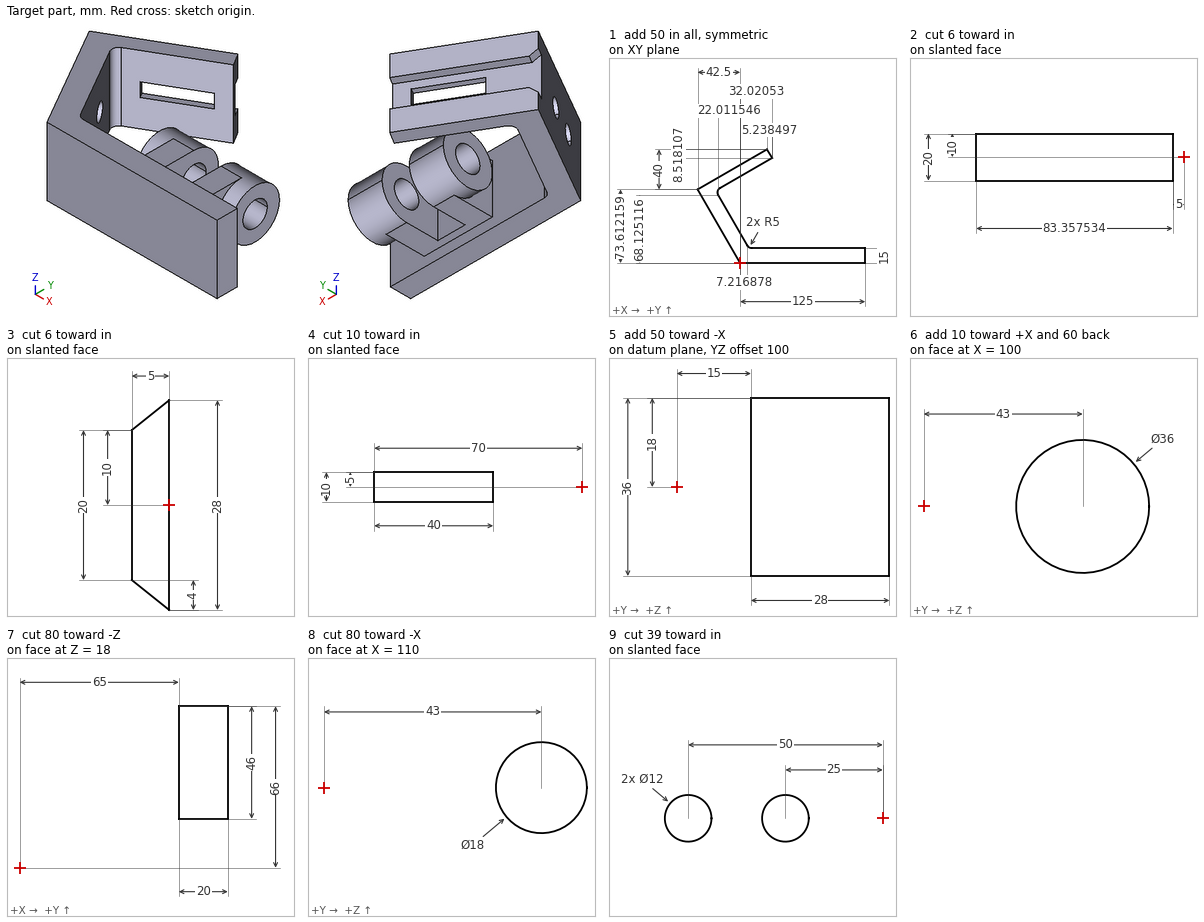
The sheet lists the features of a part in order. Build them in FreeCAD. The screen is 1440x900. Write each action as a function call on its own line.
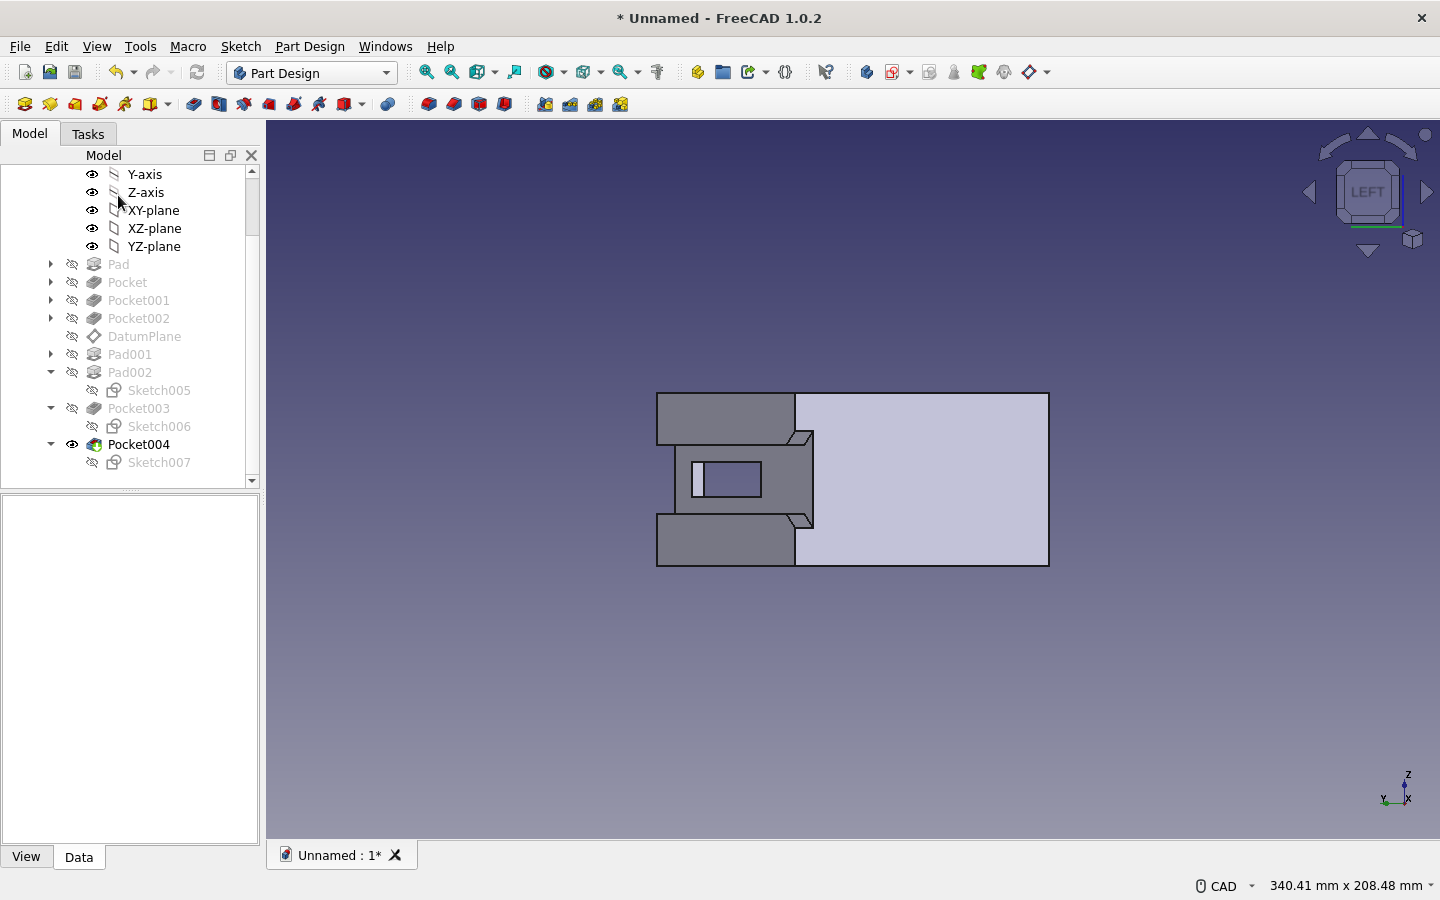
click(958, 478)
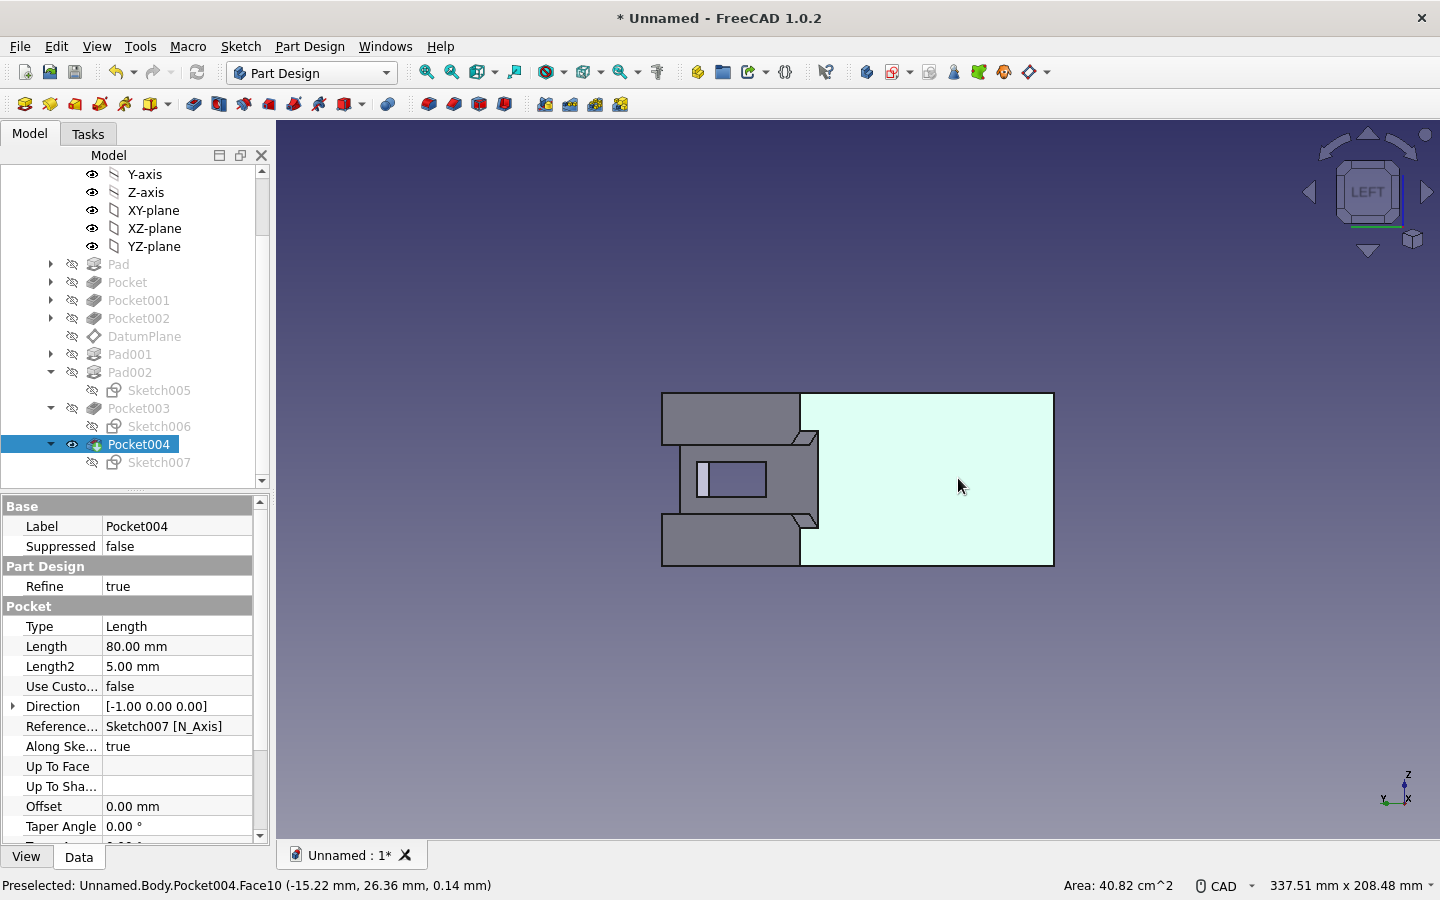
click(892, 72)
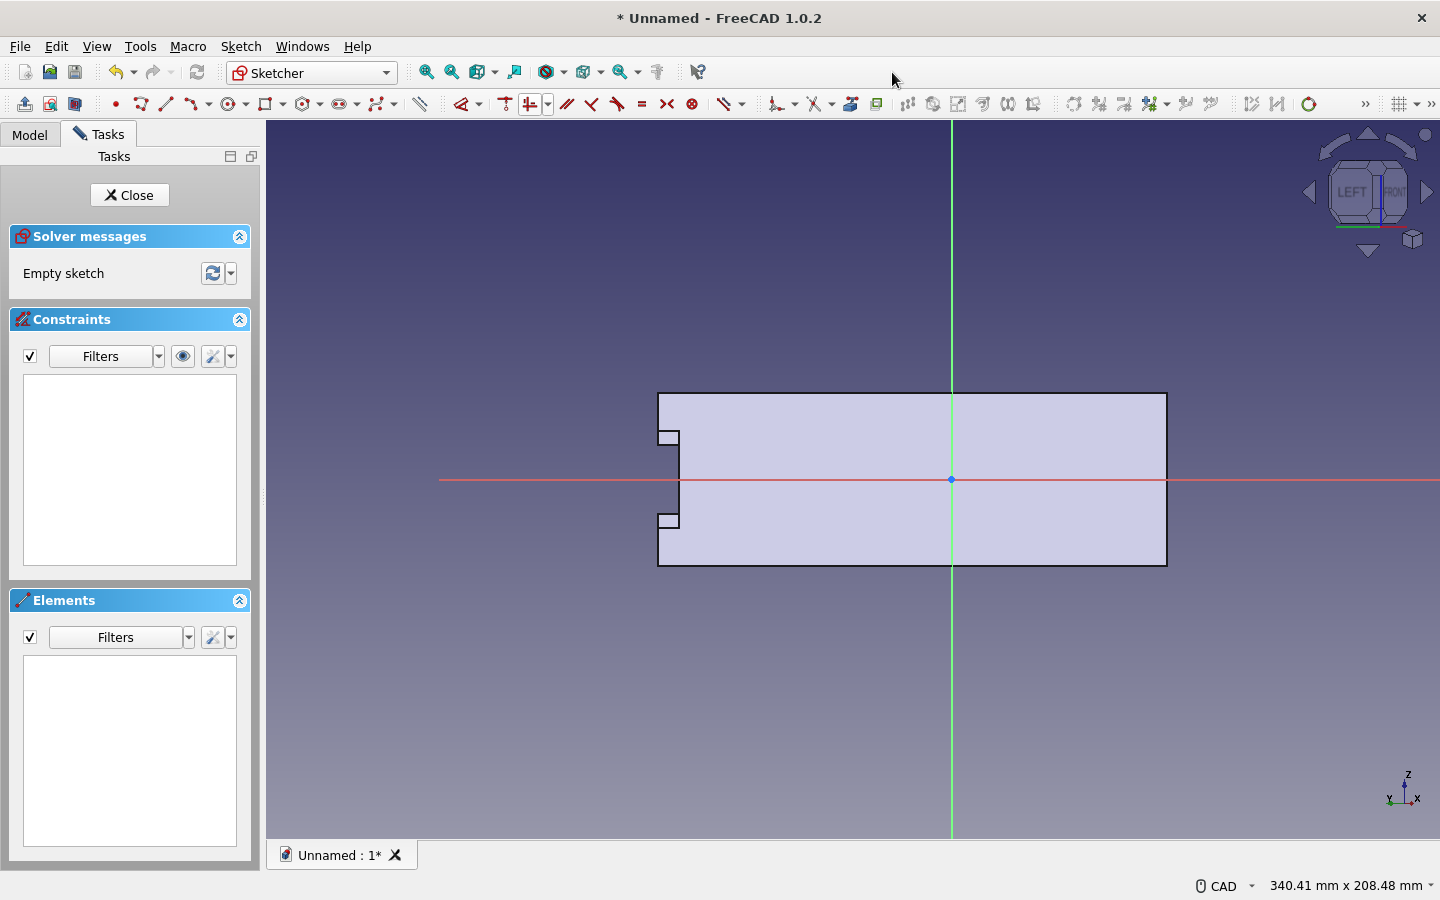
scroll(885, 479, up, 6)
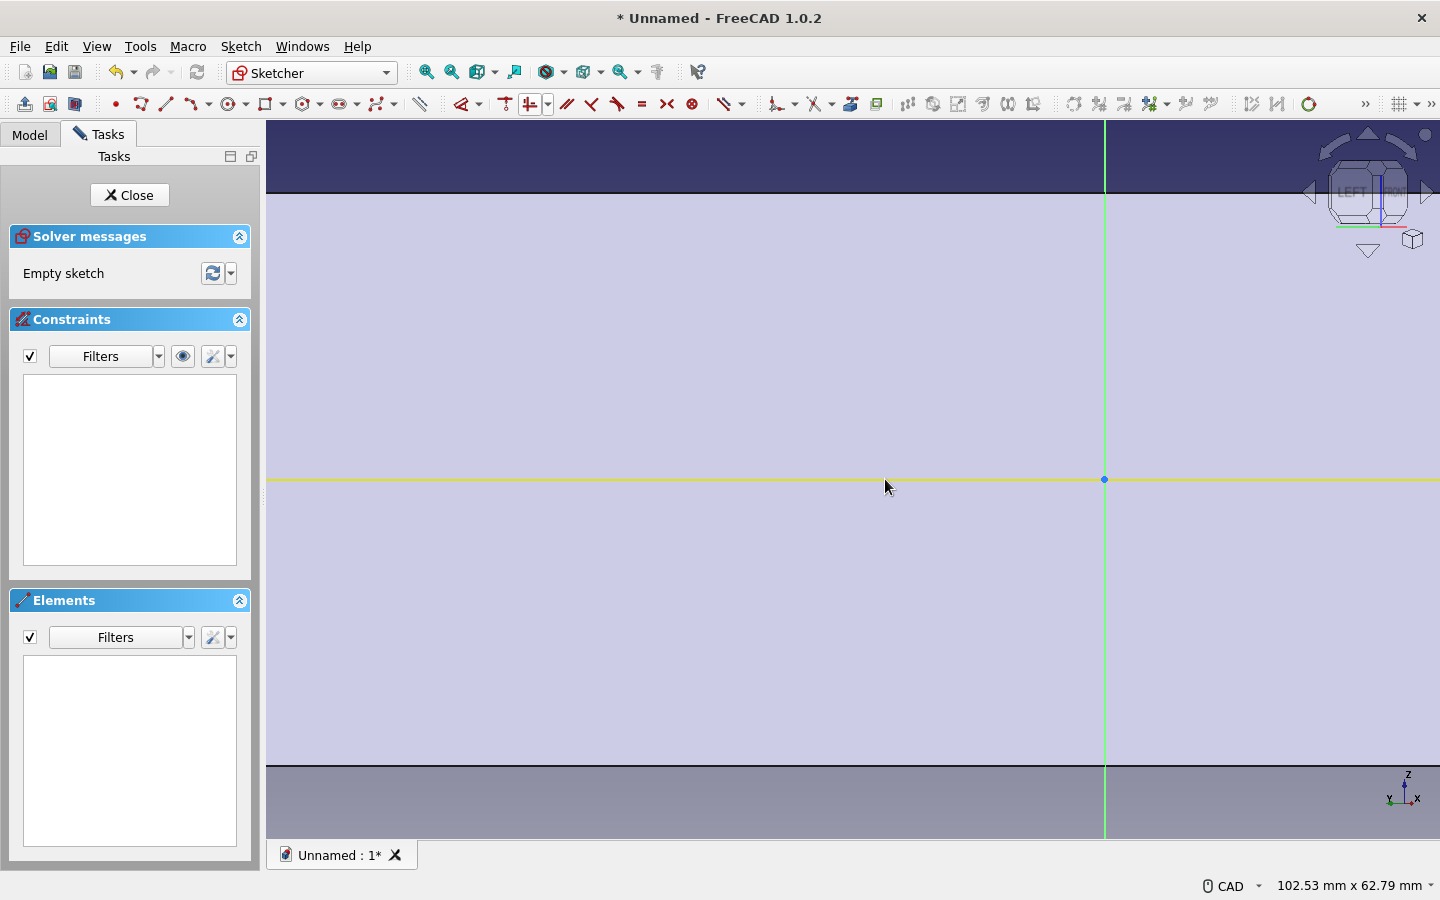
key(g)
key(c)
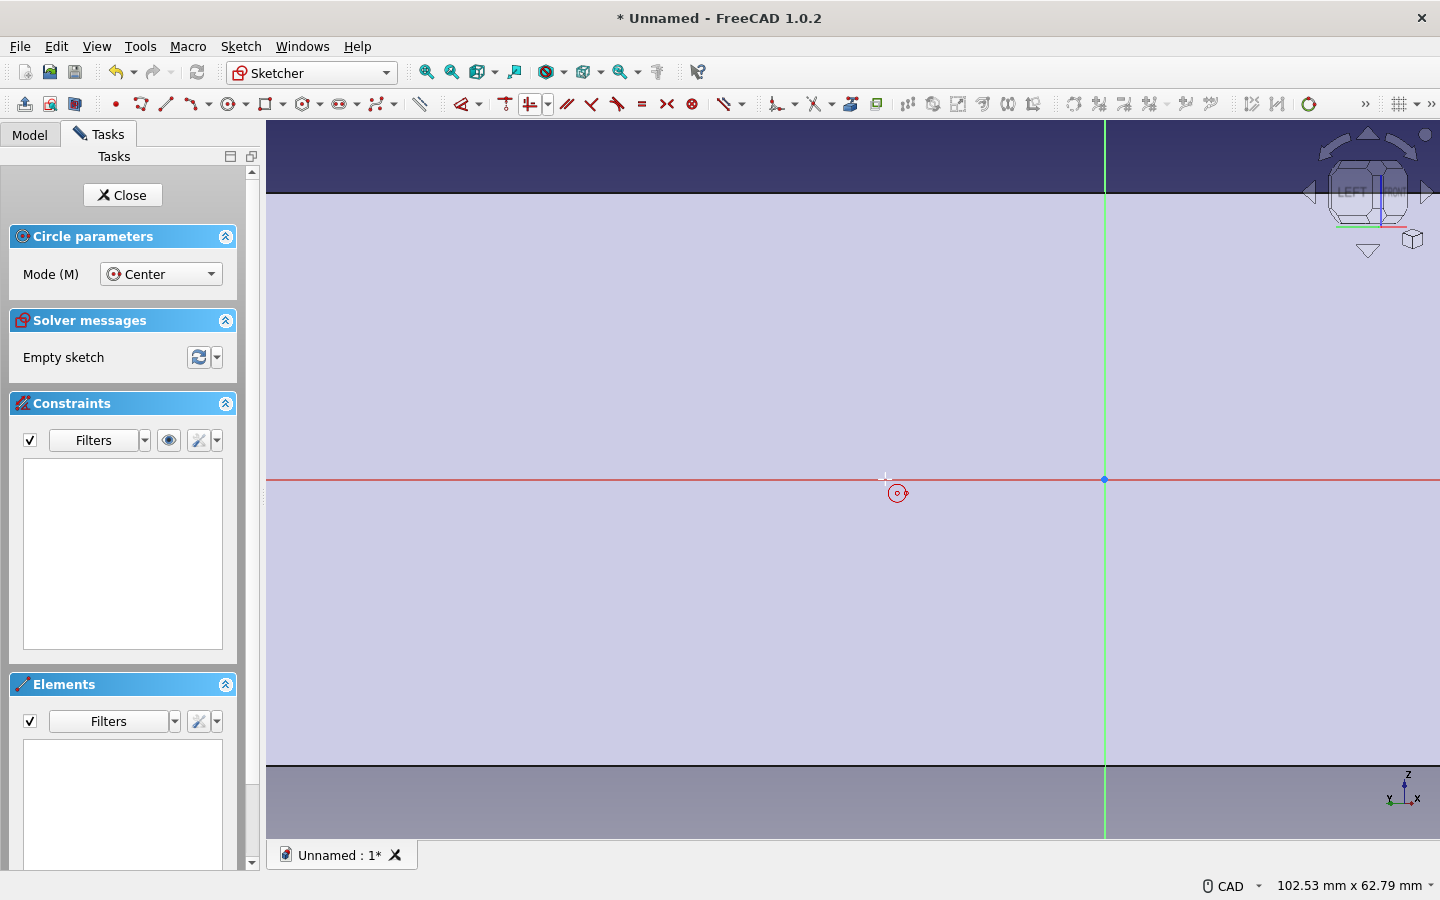
click(532, 479)
click(581, 431)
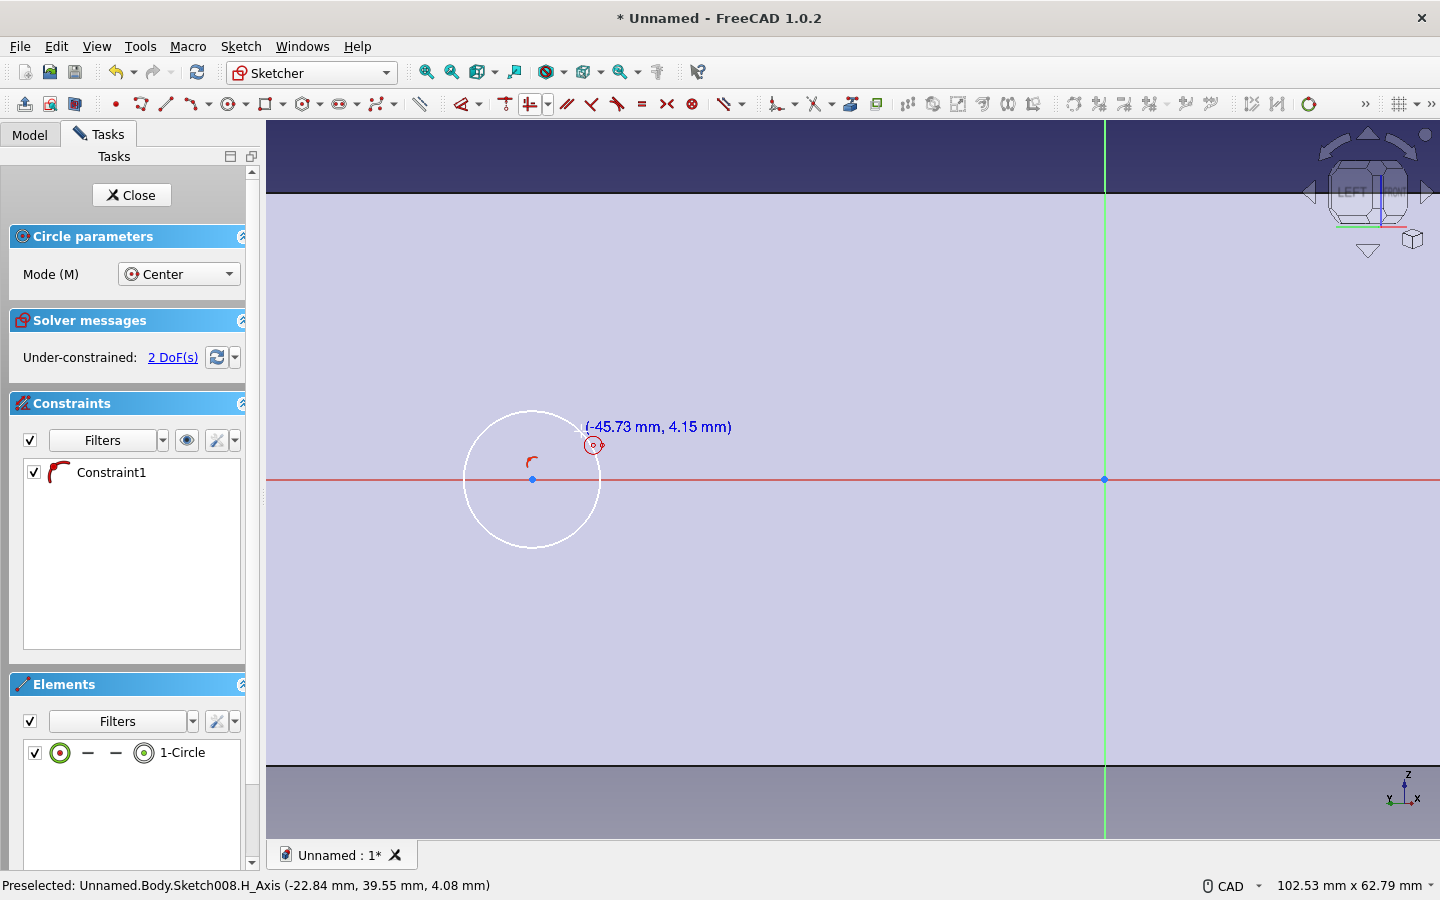
click(818, 479)
click(867, 431)
key(Escape)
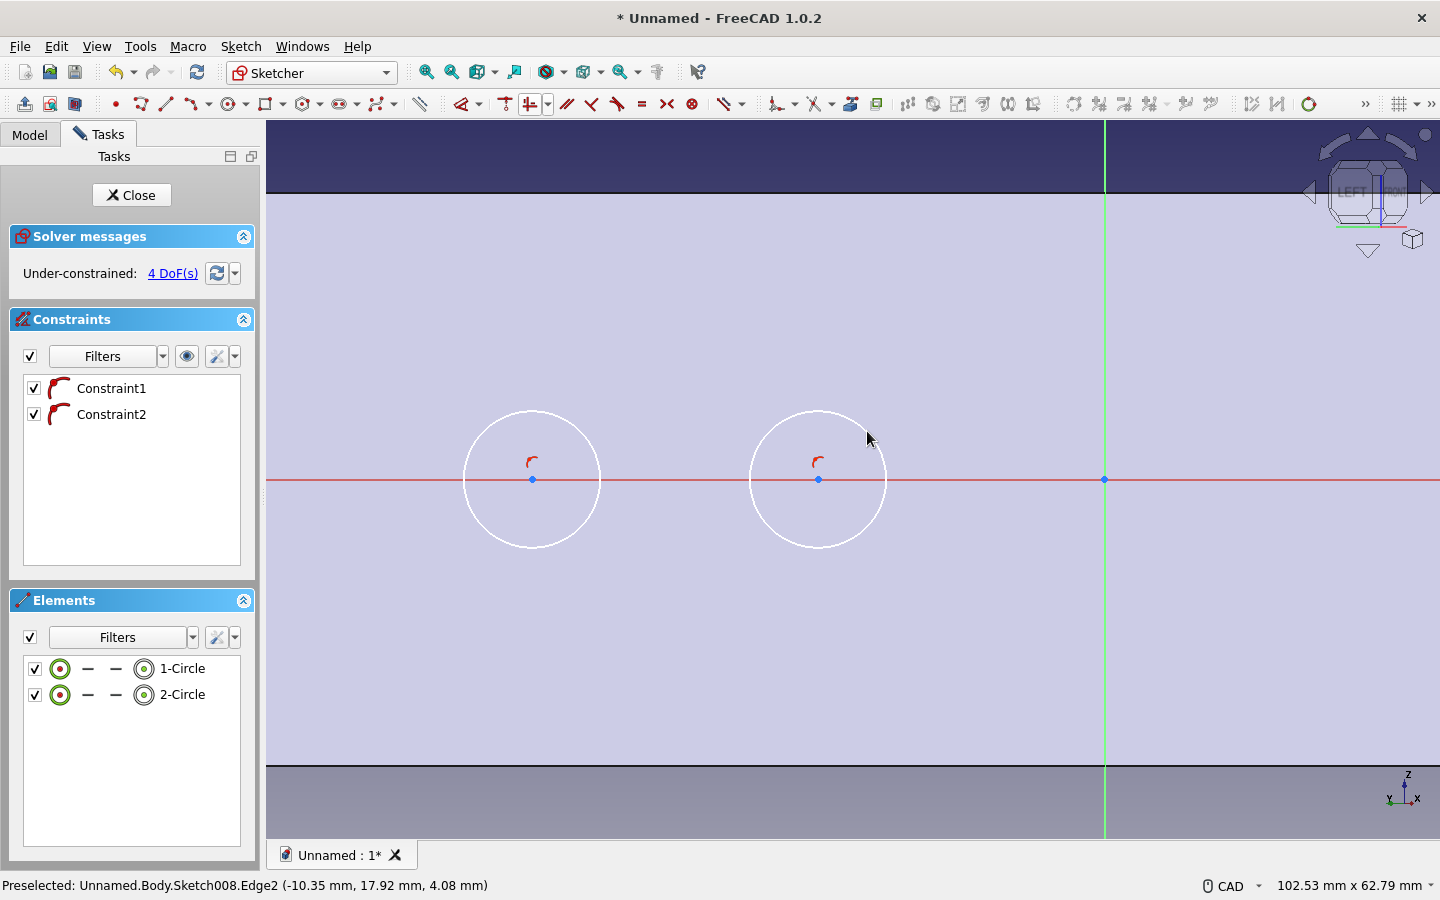
click(580, 431)